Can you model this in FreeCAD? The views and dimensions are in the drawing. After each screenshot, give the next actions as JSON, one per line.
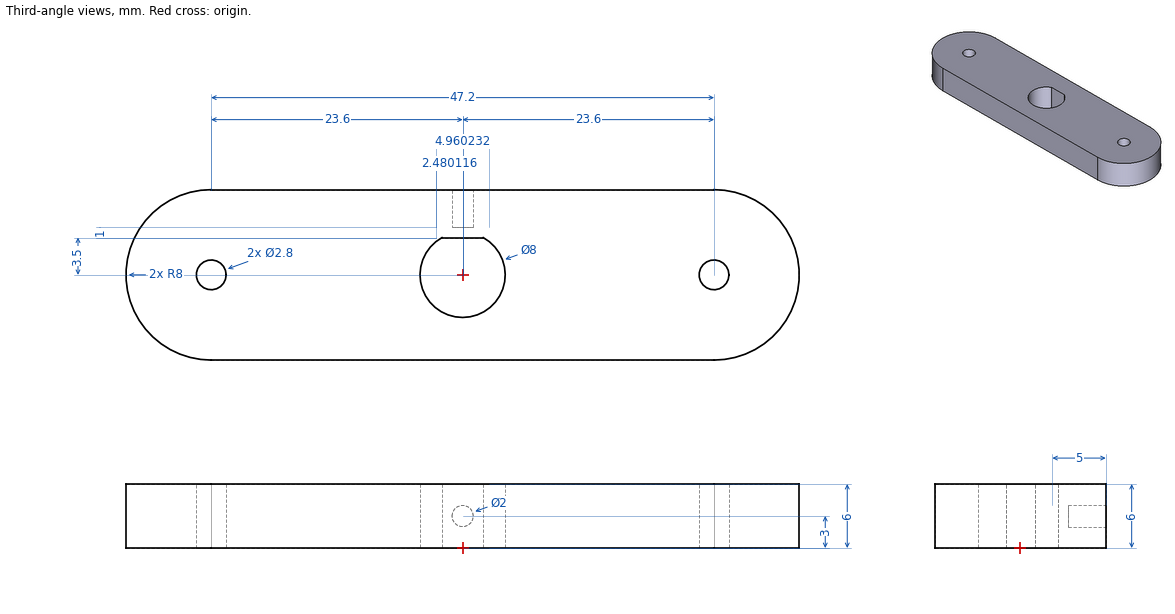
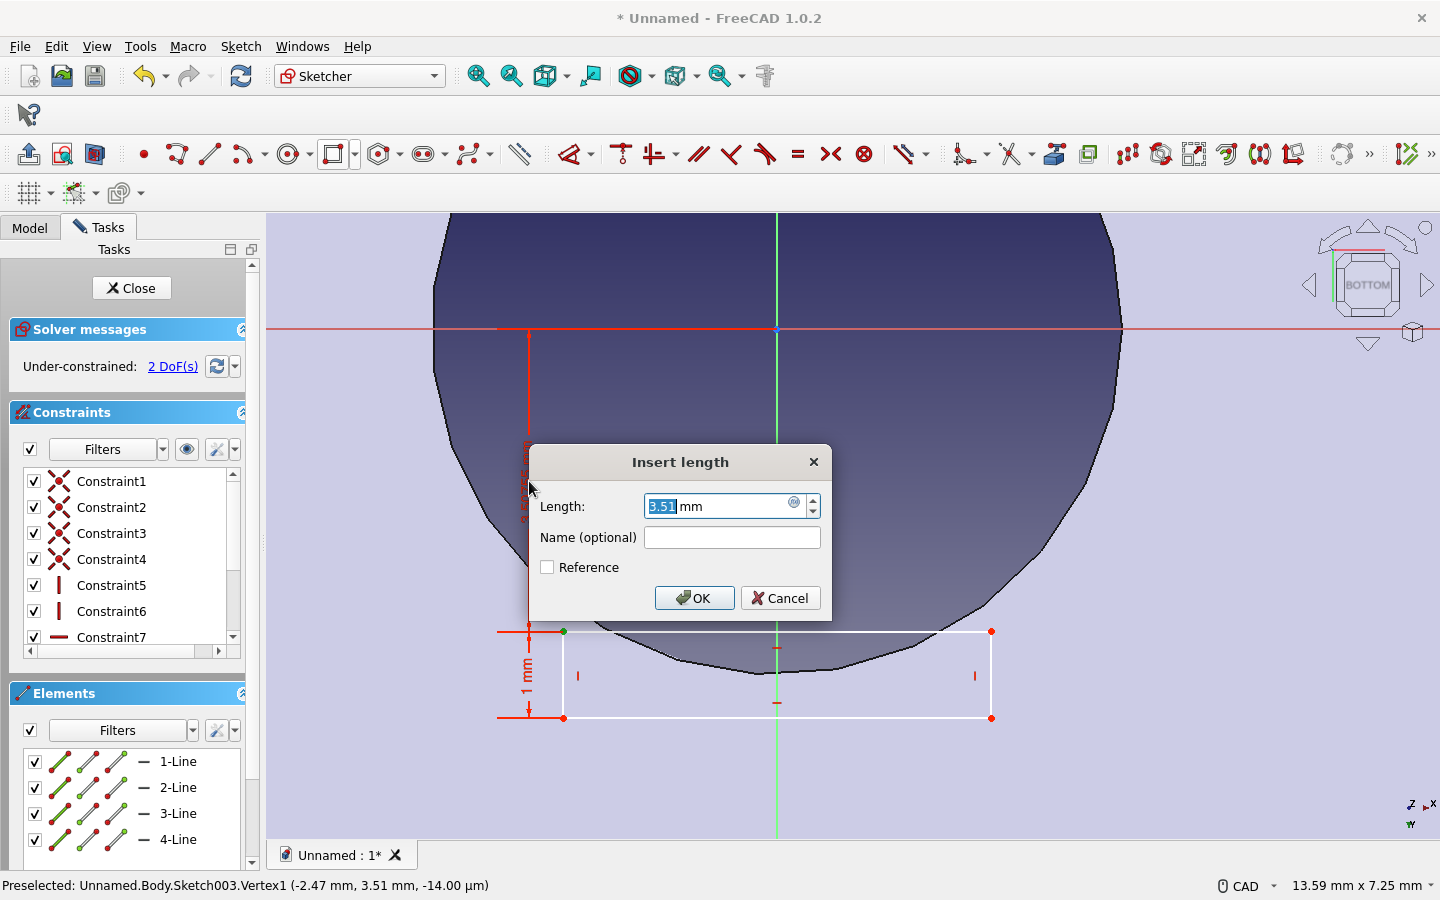
{"action": "type", "text": "3.5"}
{"action": "key", "text": "Return"}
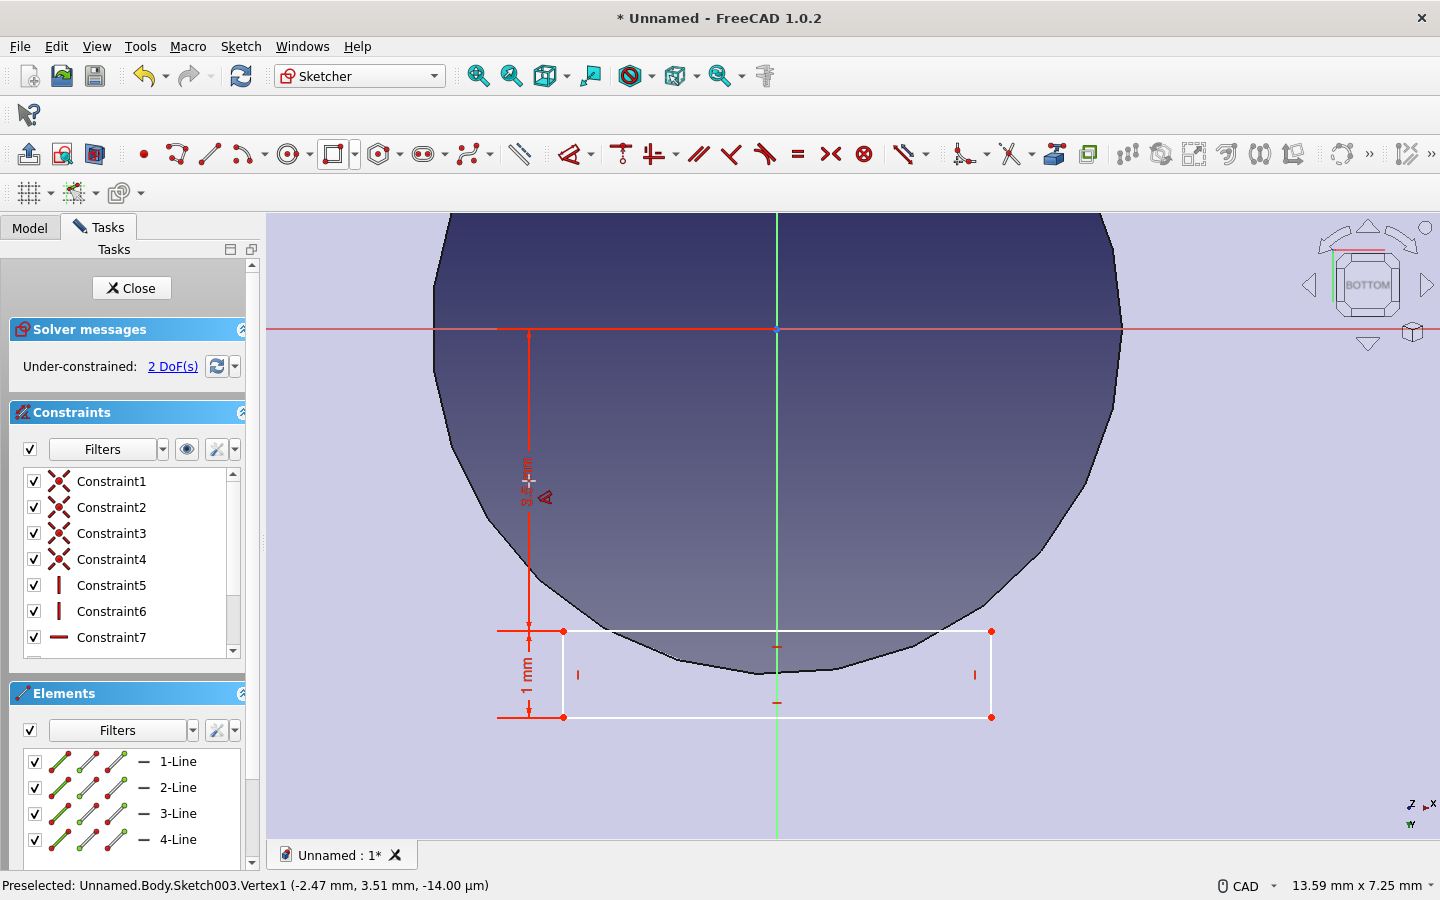
{"action": "left_click", "coordinate": [691, 718]}
{"action": "left_click", "coordinate": [679, 752]}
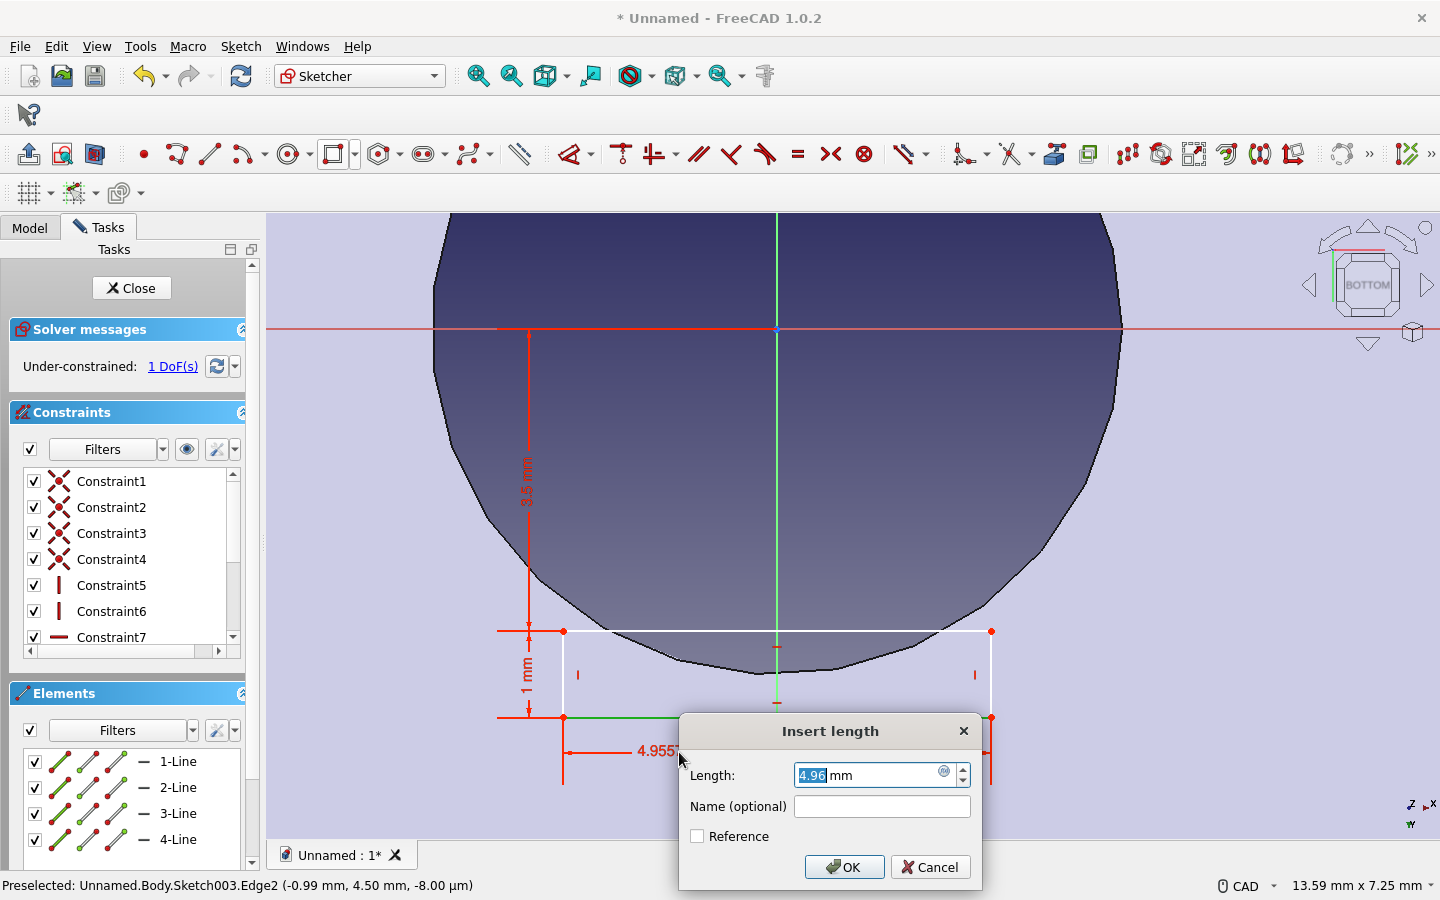
{"action": "type", "text": "4.960232"}
{"action": "key", "text": "Return"}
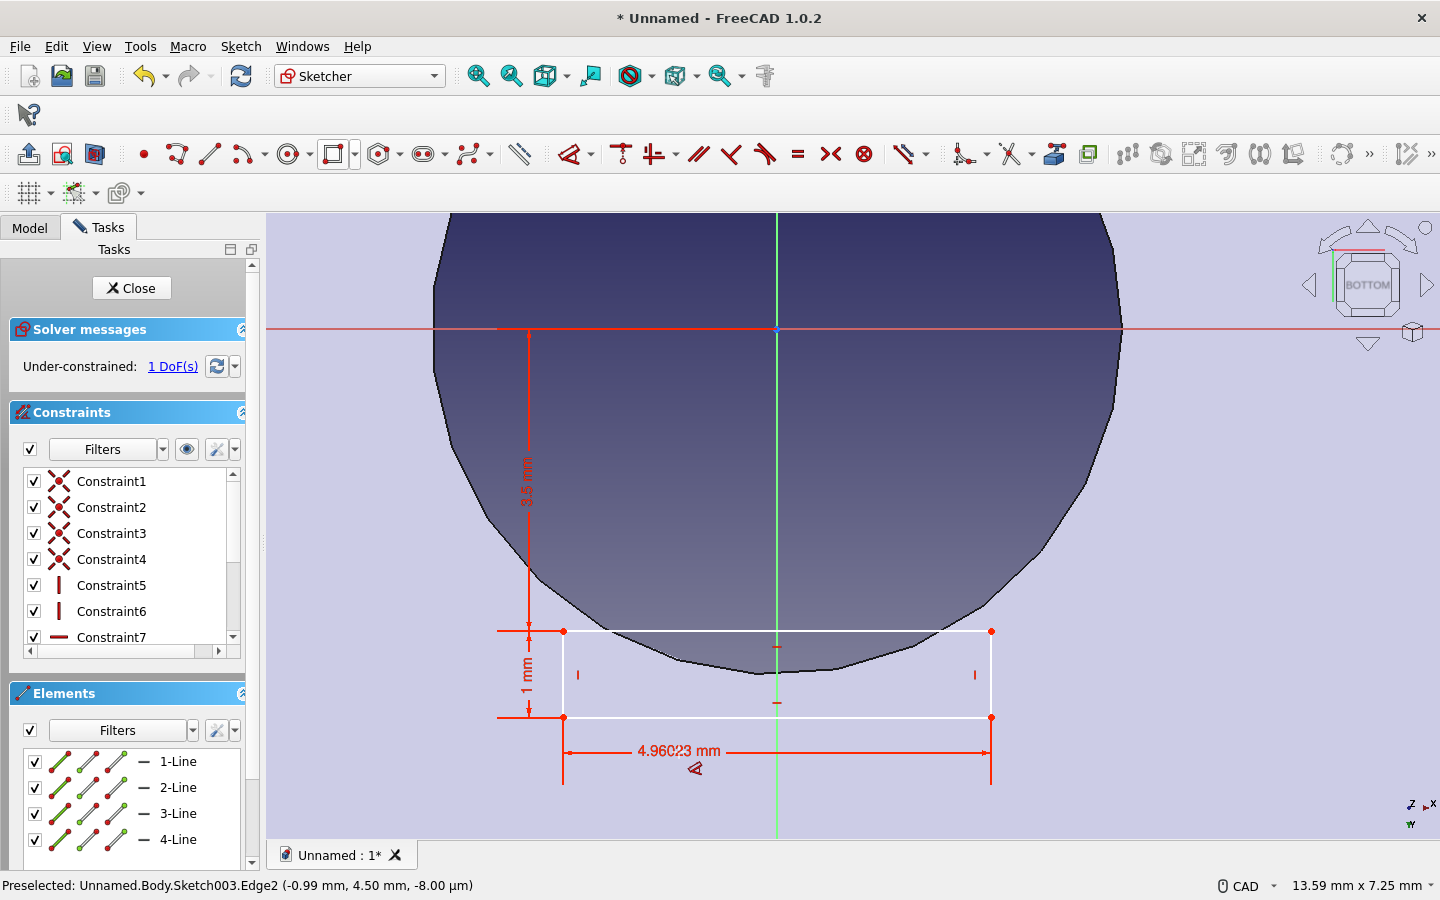
{"action": "left_click", "coordinate": [563, 631]}
{"action": "left_click", "coordinate": [670, 295]}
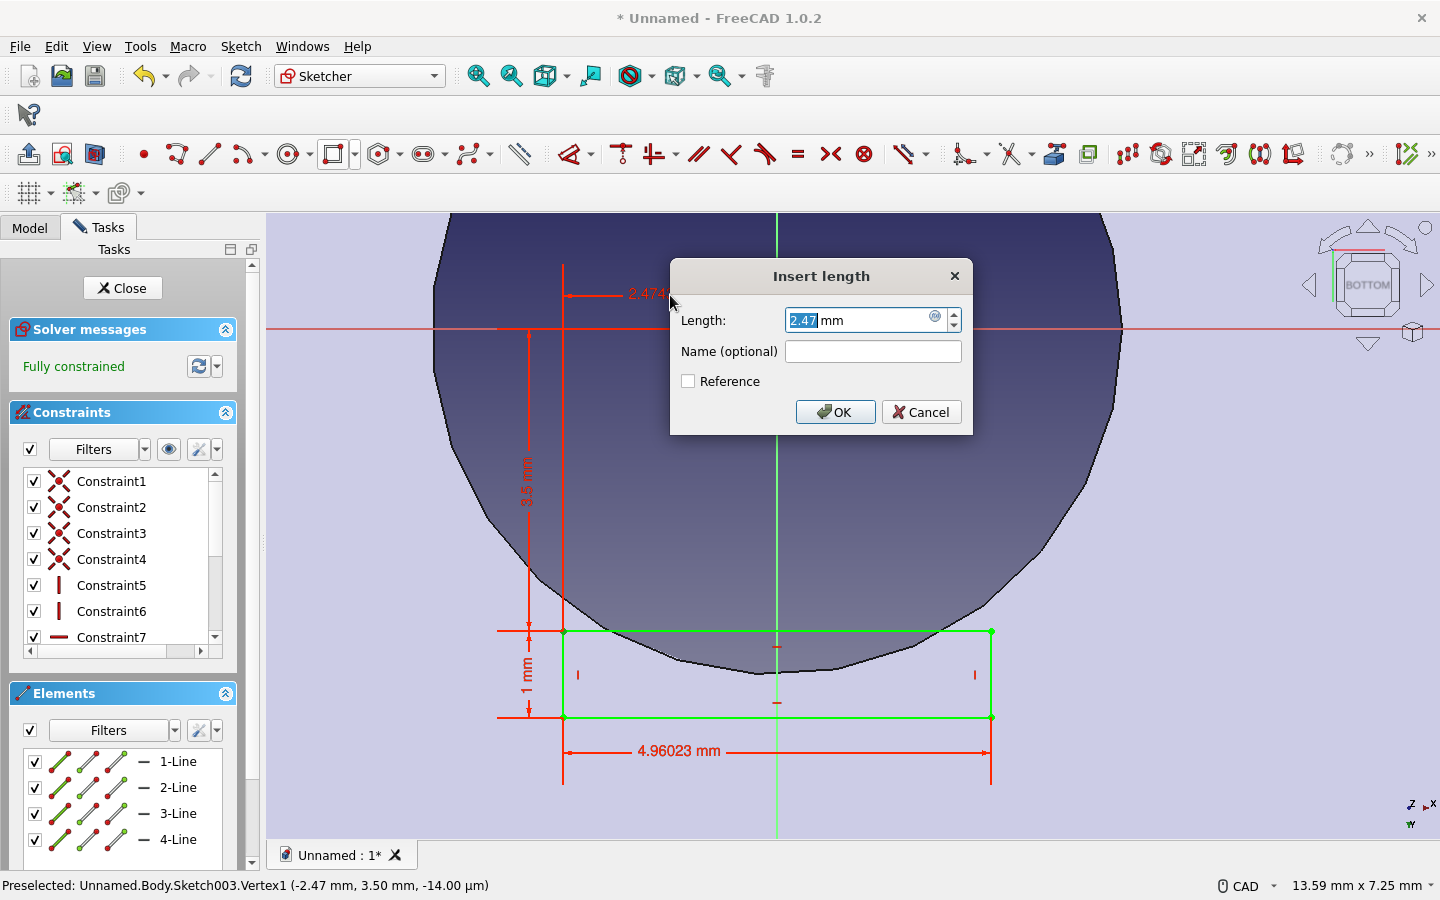
{"action": "type", "text": "2.480116"}
{"action": "key", "text": "Return"}
{"action": "key", "text": "Escape"}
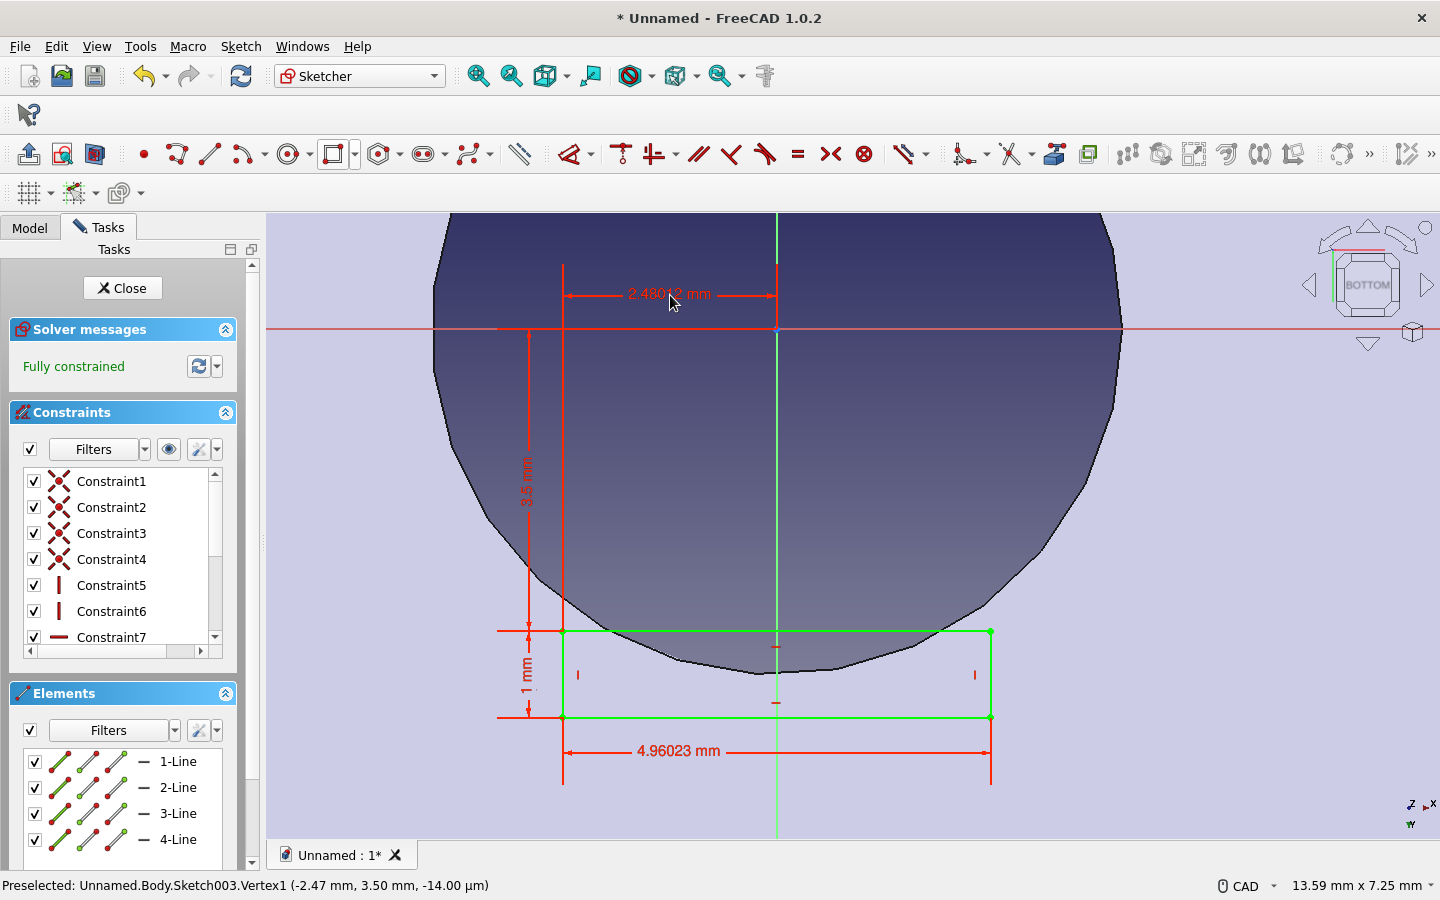
{"action": "left_click", "coordinate": [123, 288]}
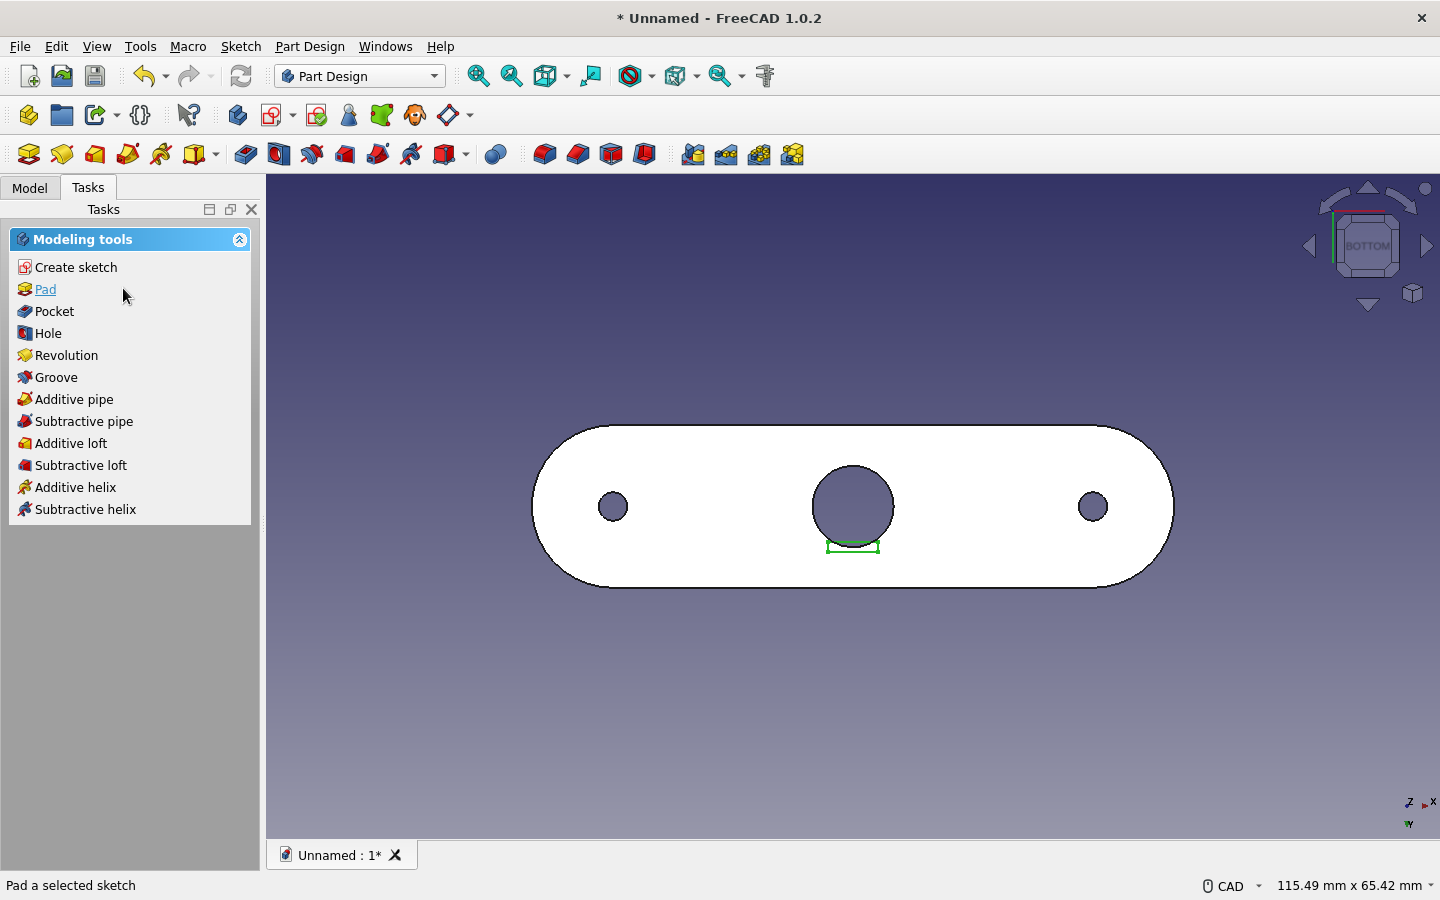
{"action": "left_click", "coordinate": [29, 154]}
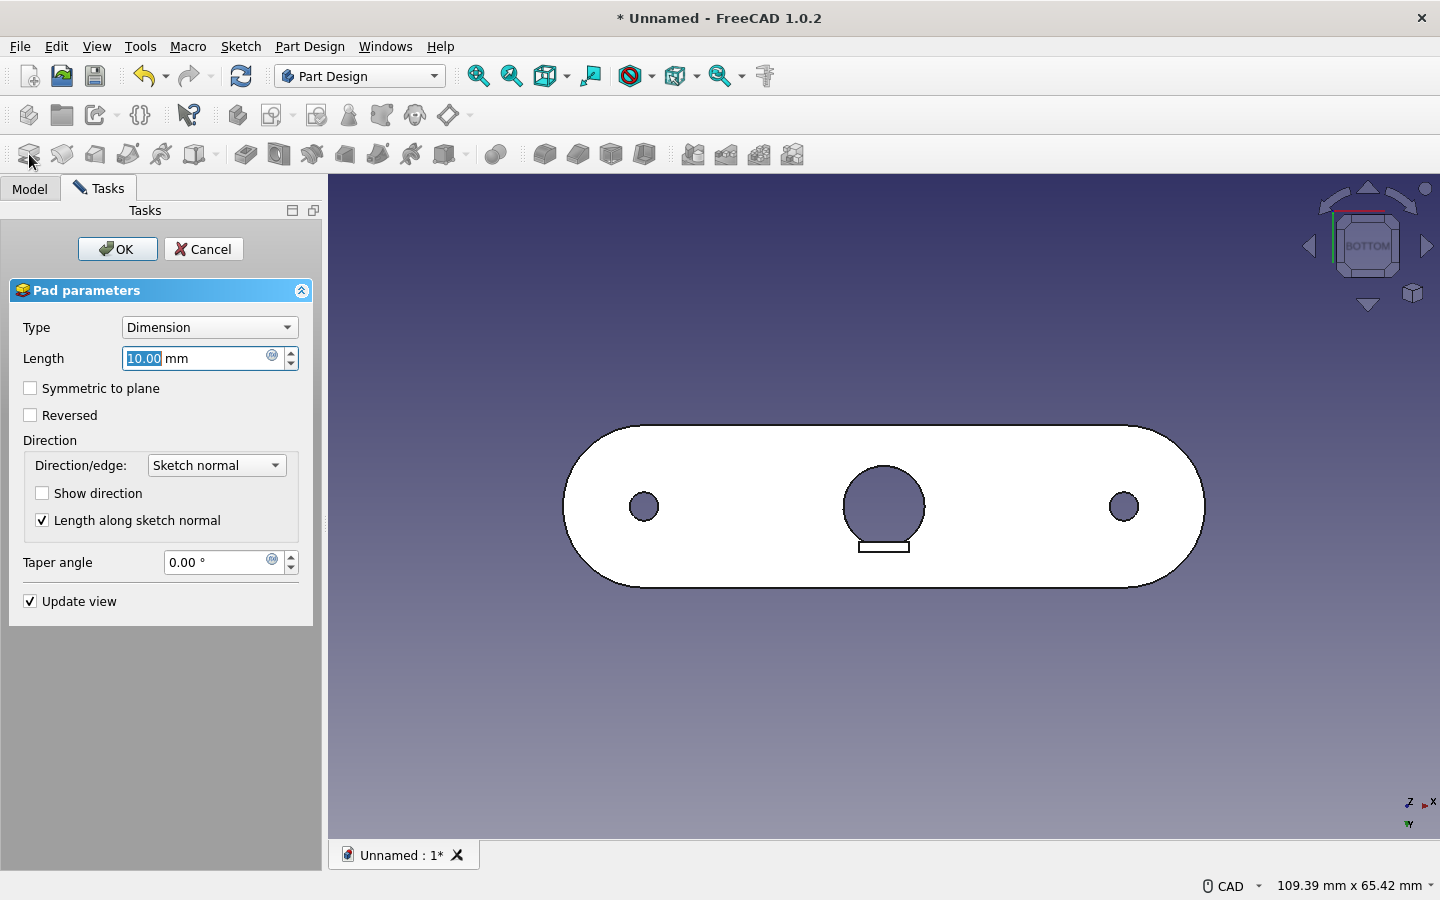
{"action": "type", "text": "6"}
{"action": "key", "text": "Tab"}